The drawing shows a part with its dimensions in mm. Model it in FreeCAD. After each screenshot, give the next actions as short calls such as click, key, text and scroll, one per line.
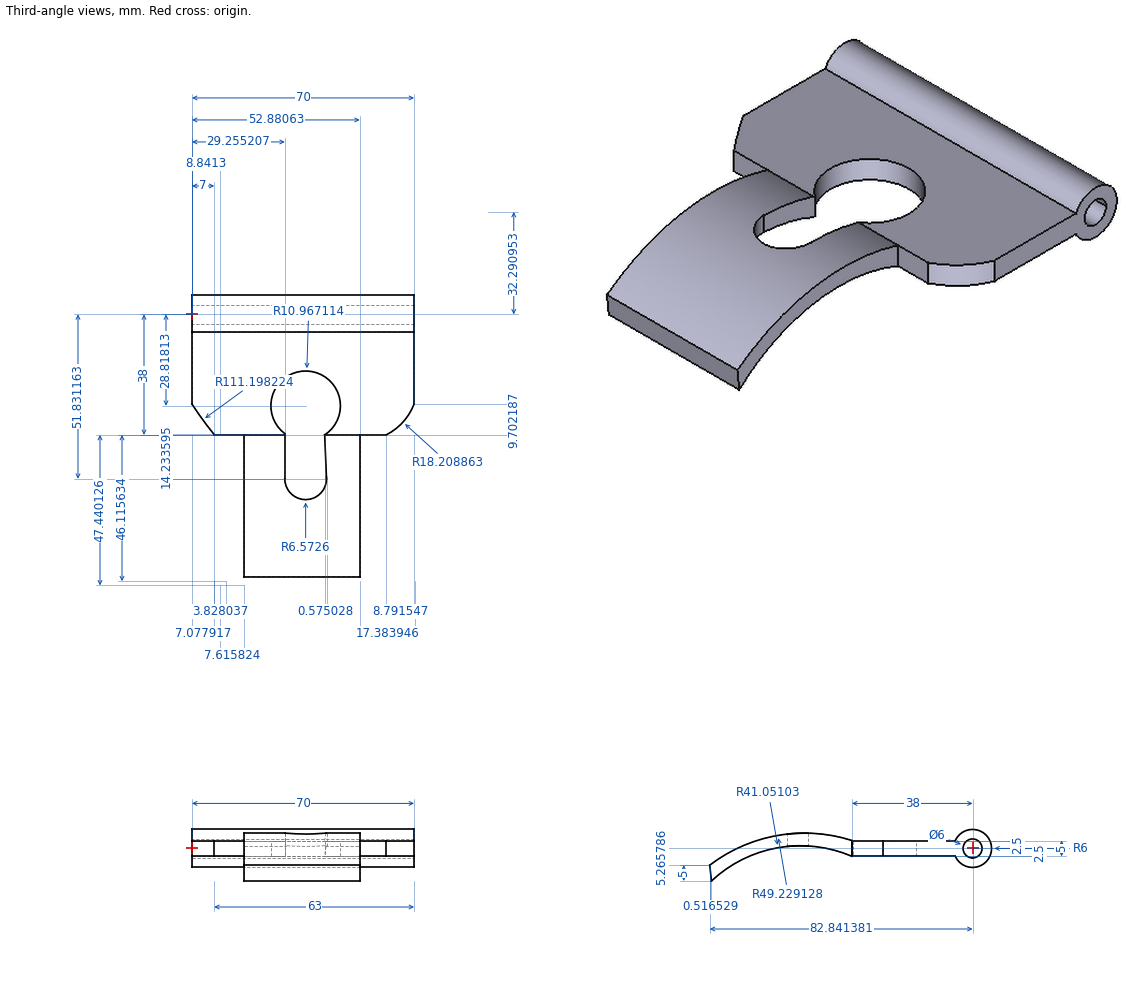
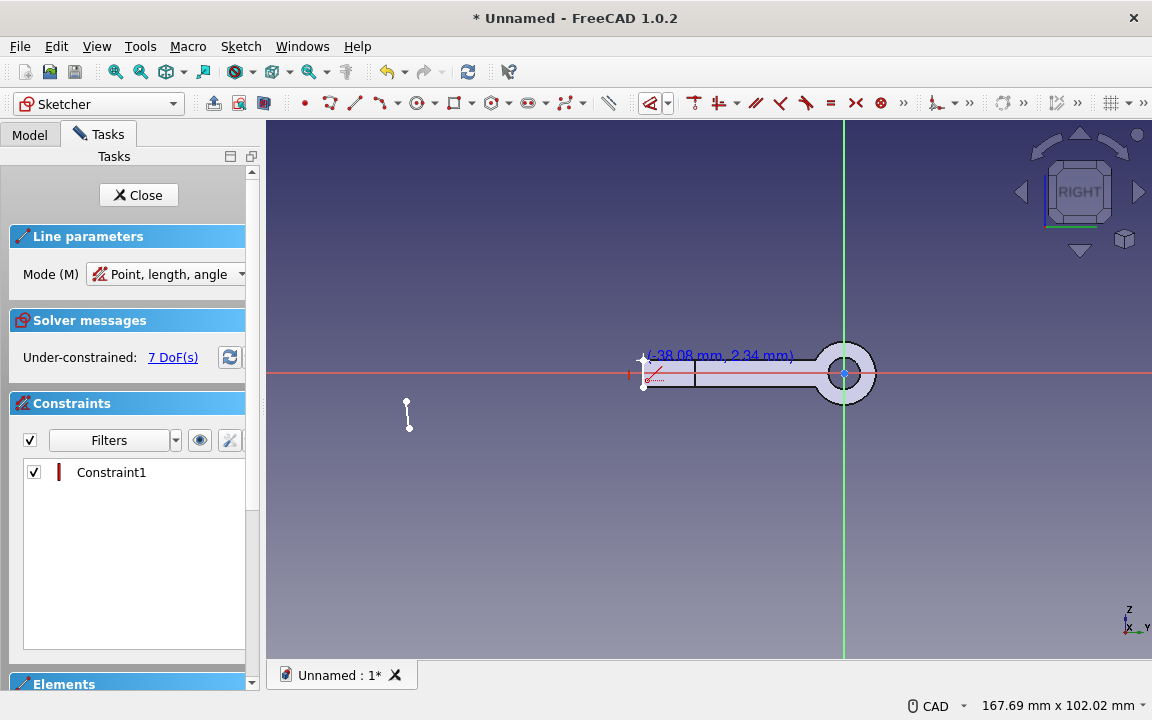
click(380, 104)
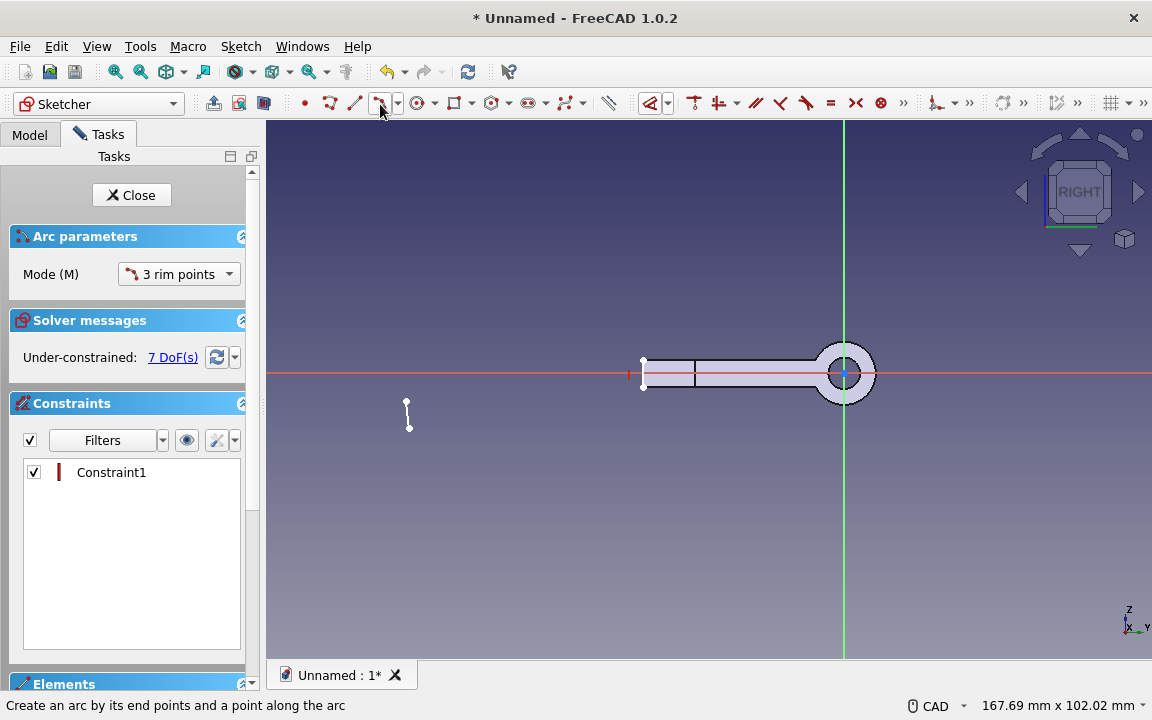
click(409, 429)
click(643, 388)
click(472, 386)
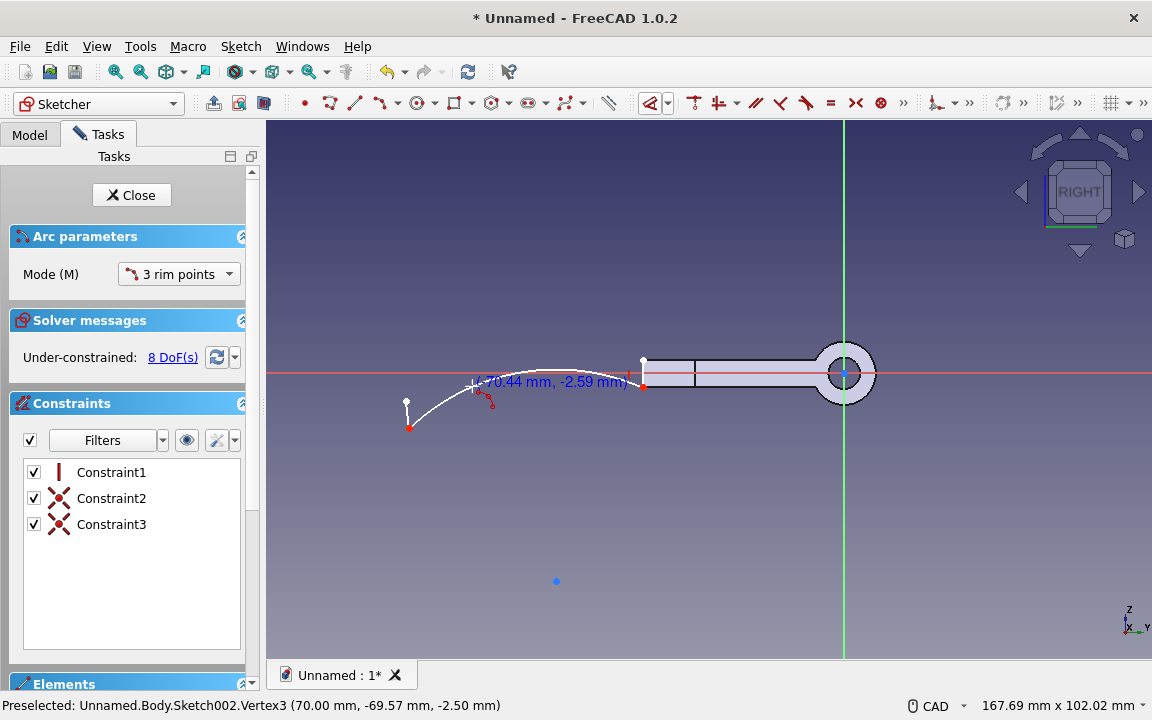
click(643, 361)
click(406, 402)
click(520, 352)
key(Escape)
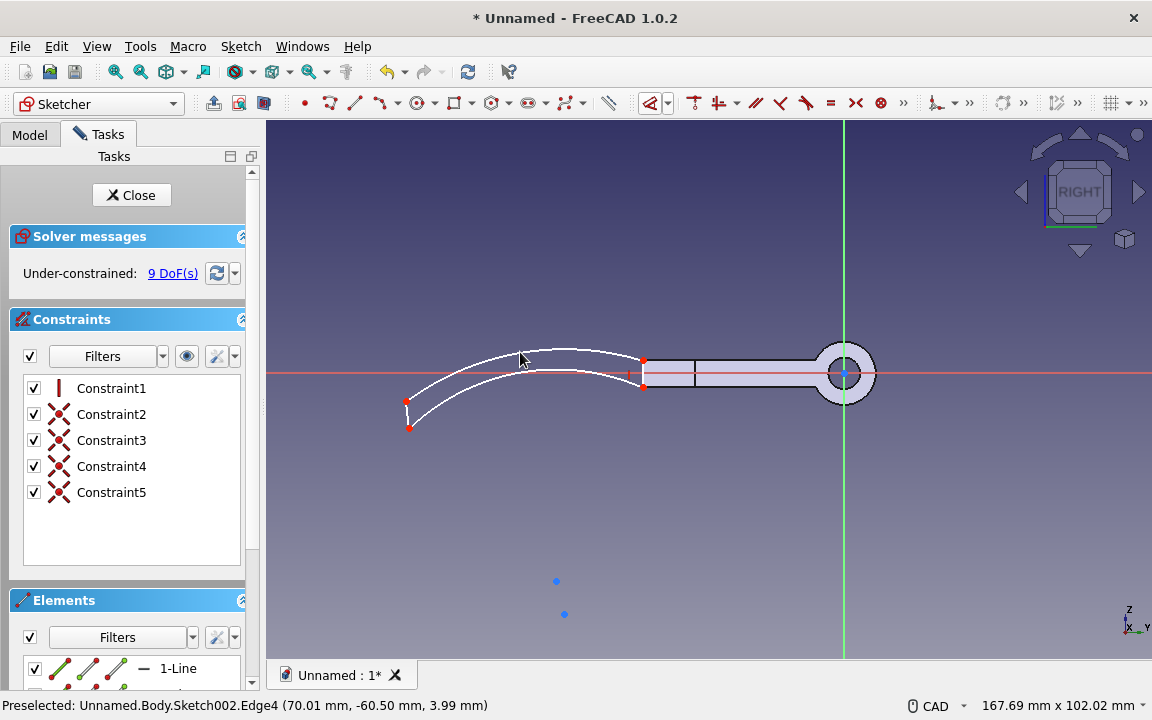
click(570, 370)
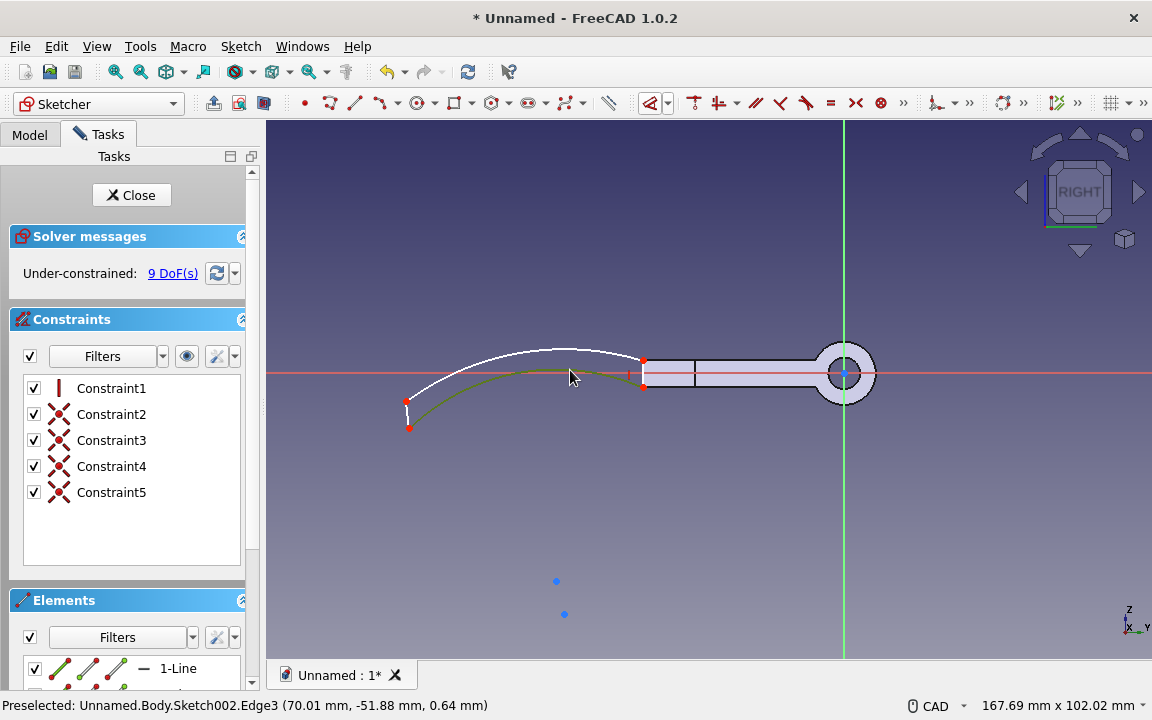
click(668, 104)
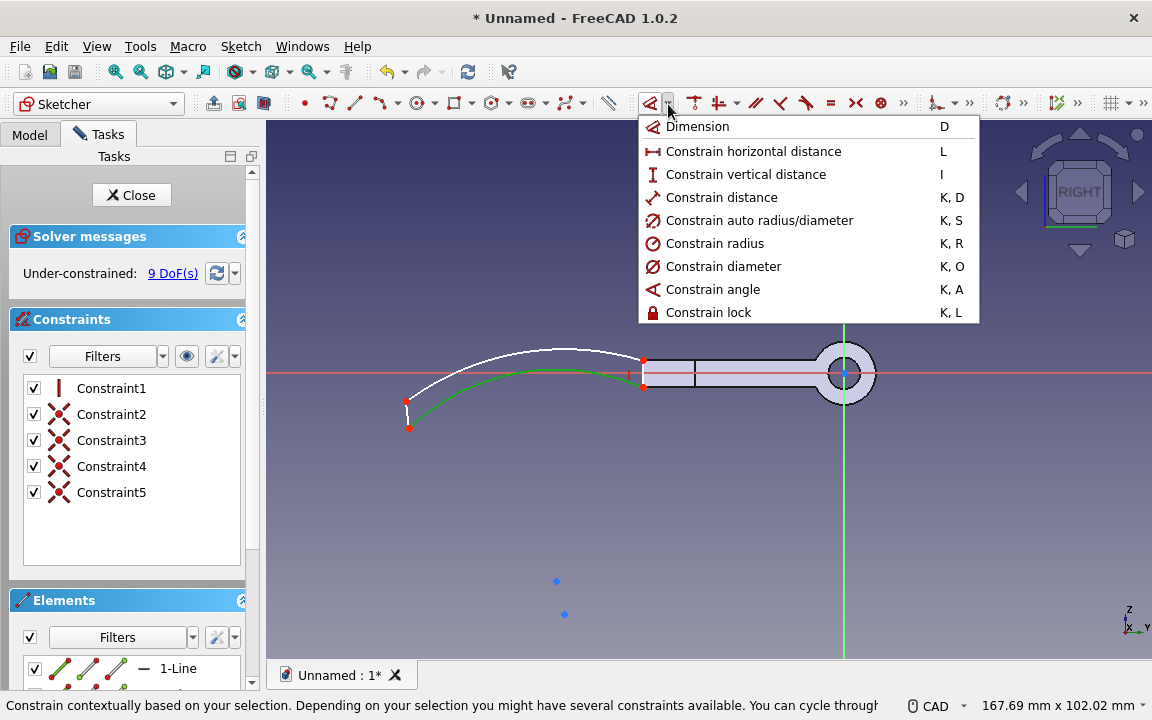
click(809, 244)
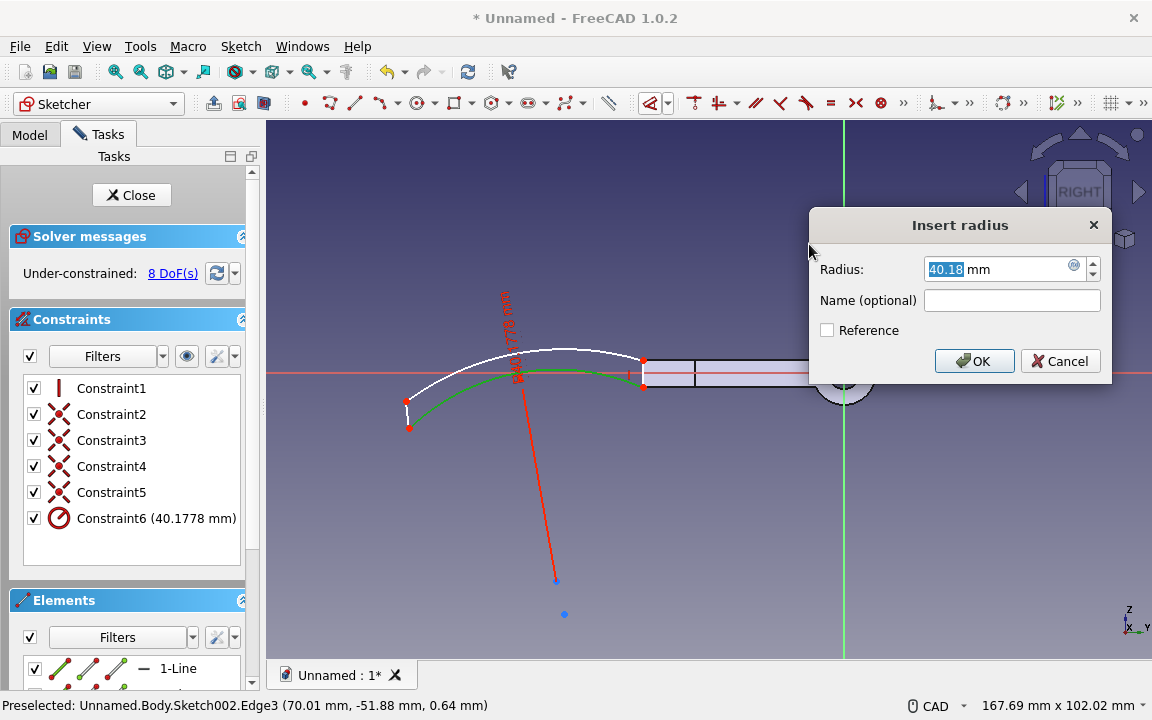
text(41.05103)
key(Return)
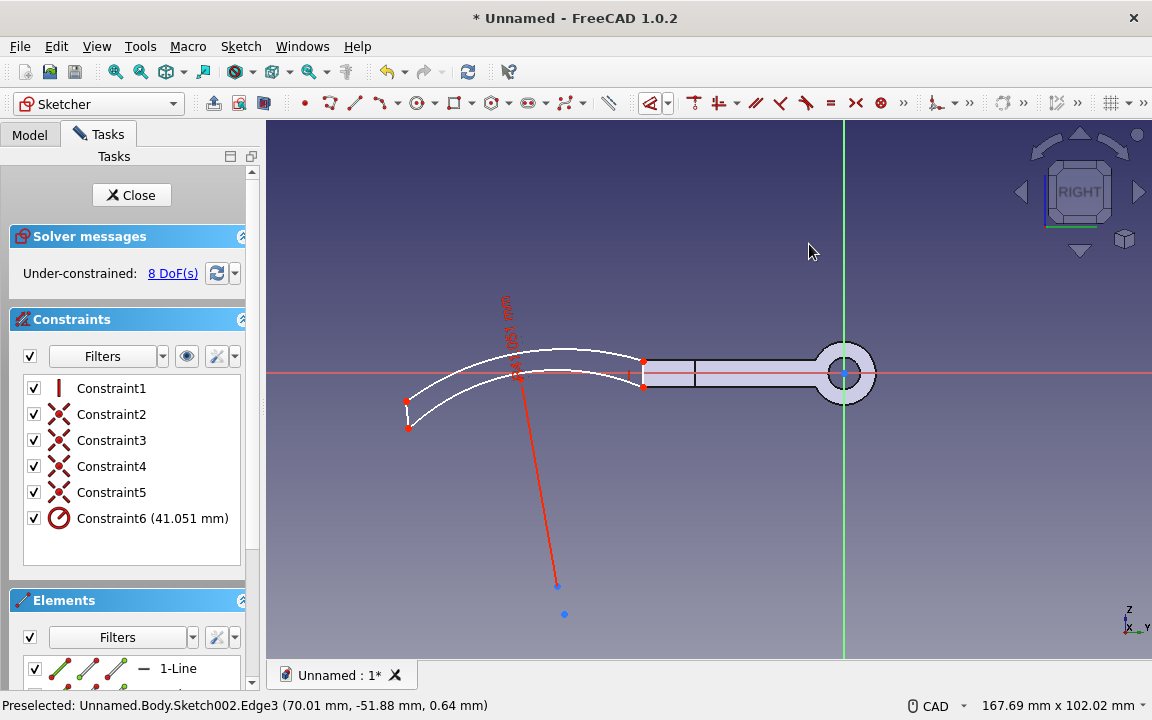
click(569, 349)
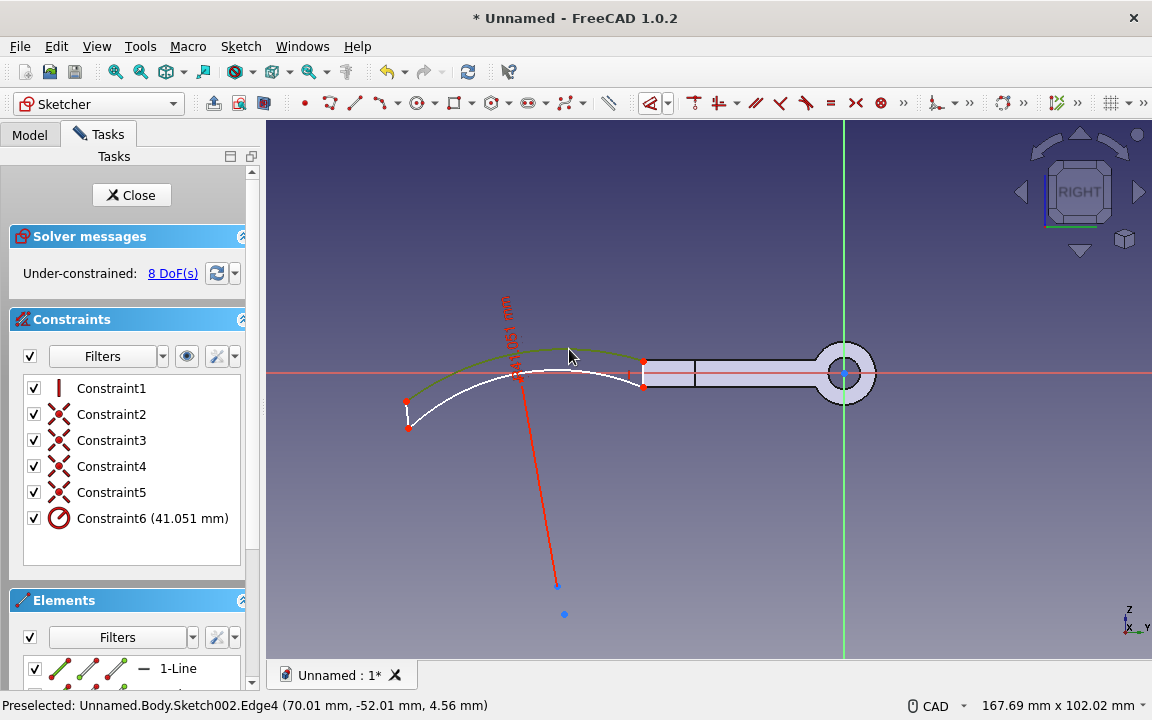
click(668, 104)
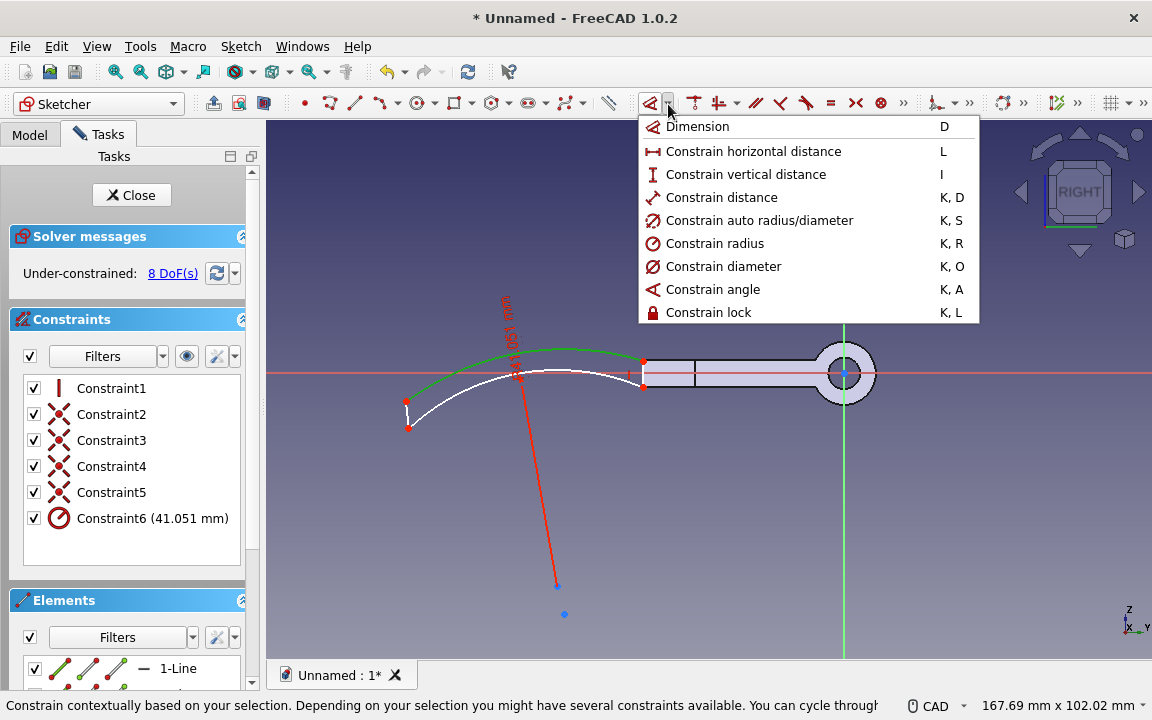
click(809, 244)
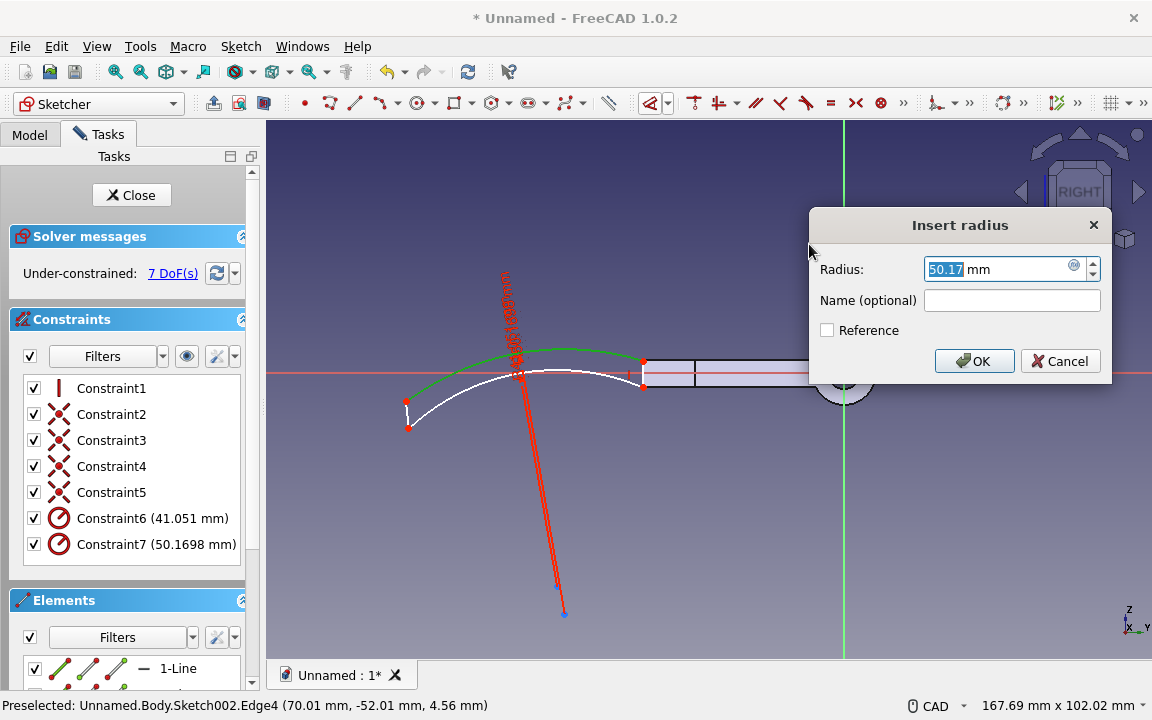
text(49.229128)
key(Return)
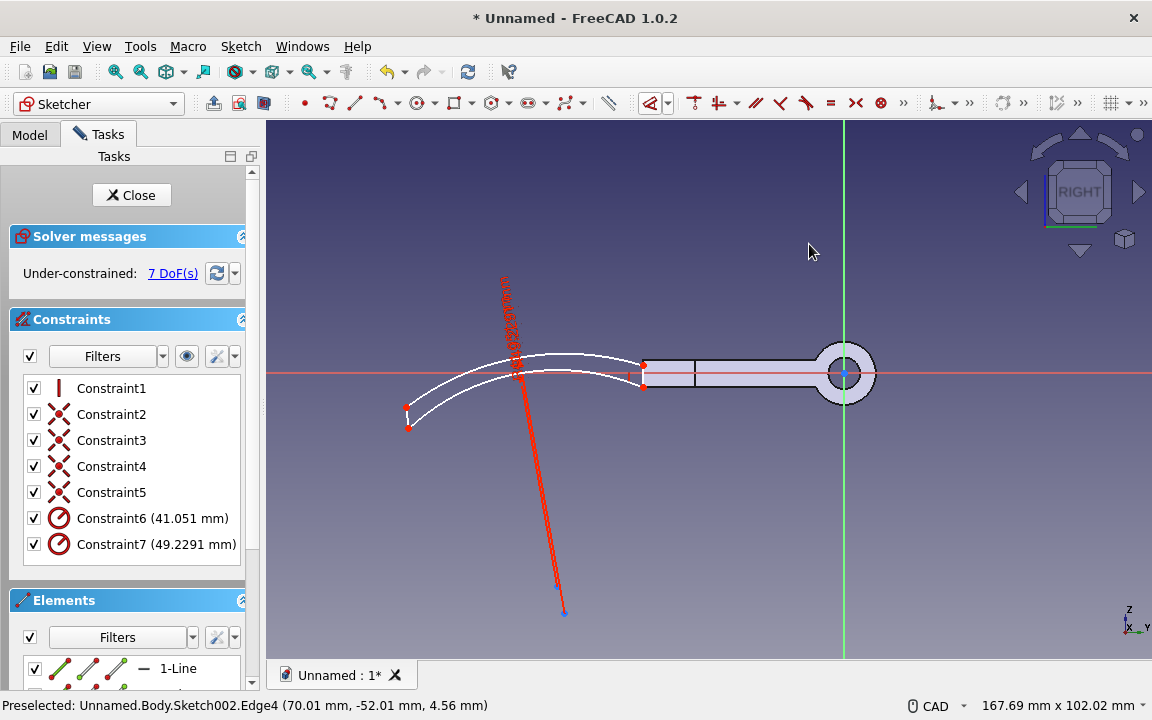
scroll(643, 377, up, 3)